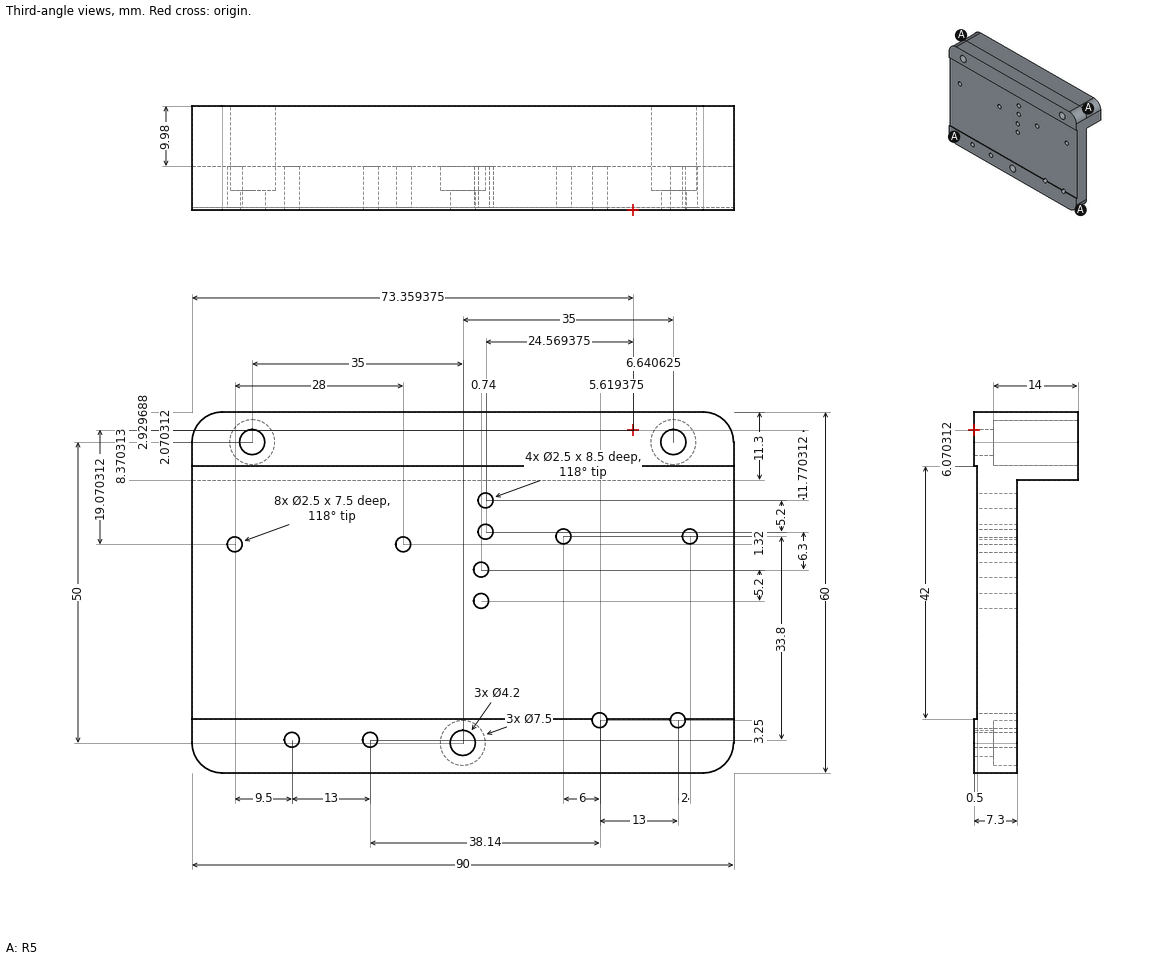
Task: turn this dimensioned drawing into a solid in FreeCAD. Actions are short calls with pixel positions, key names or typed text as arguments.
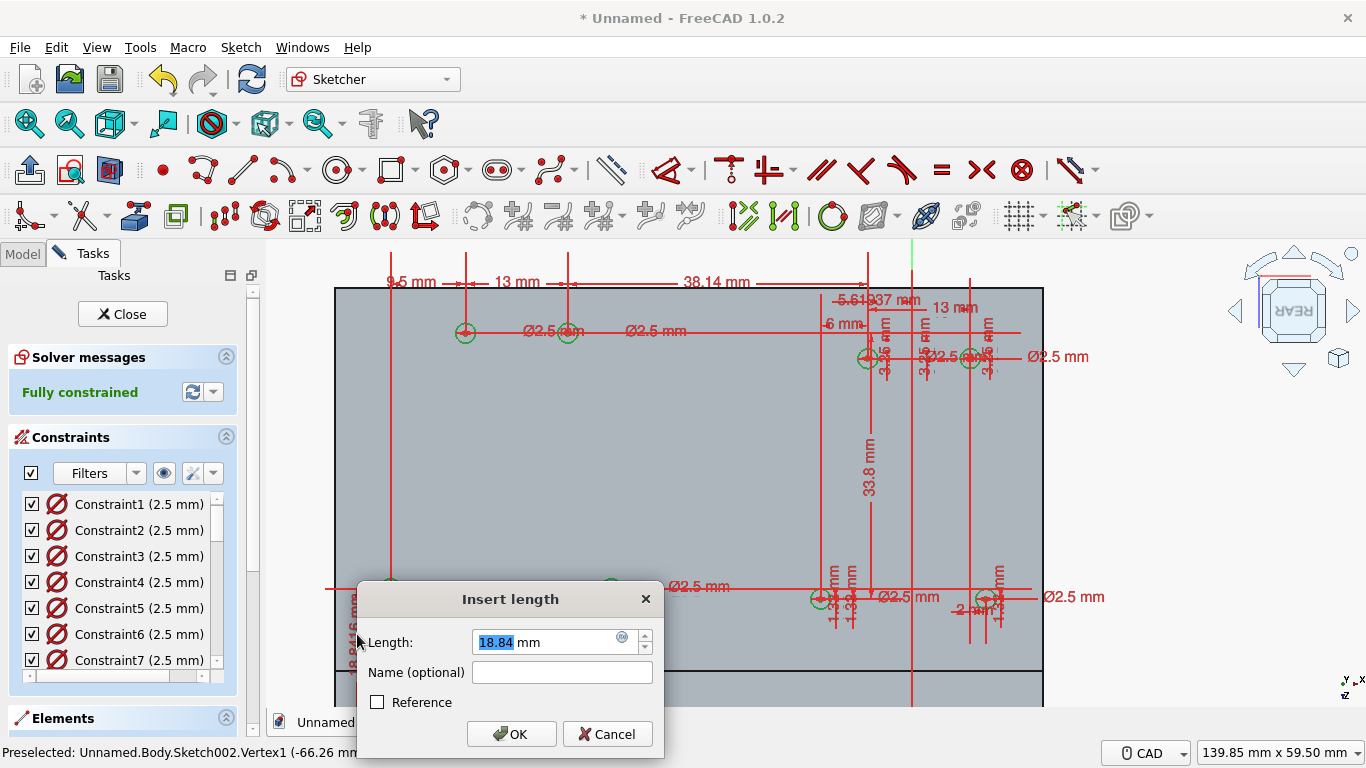
text(19.070312)
key(Return)
key(Escape)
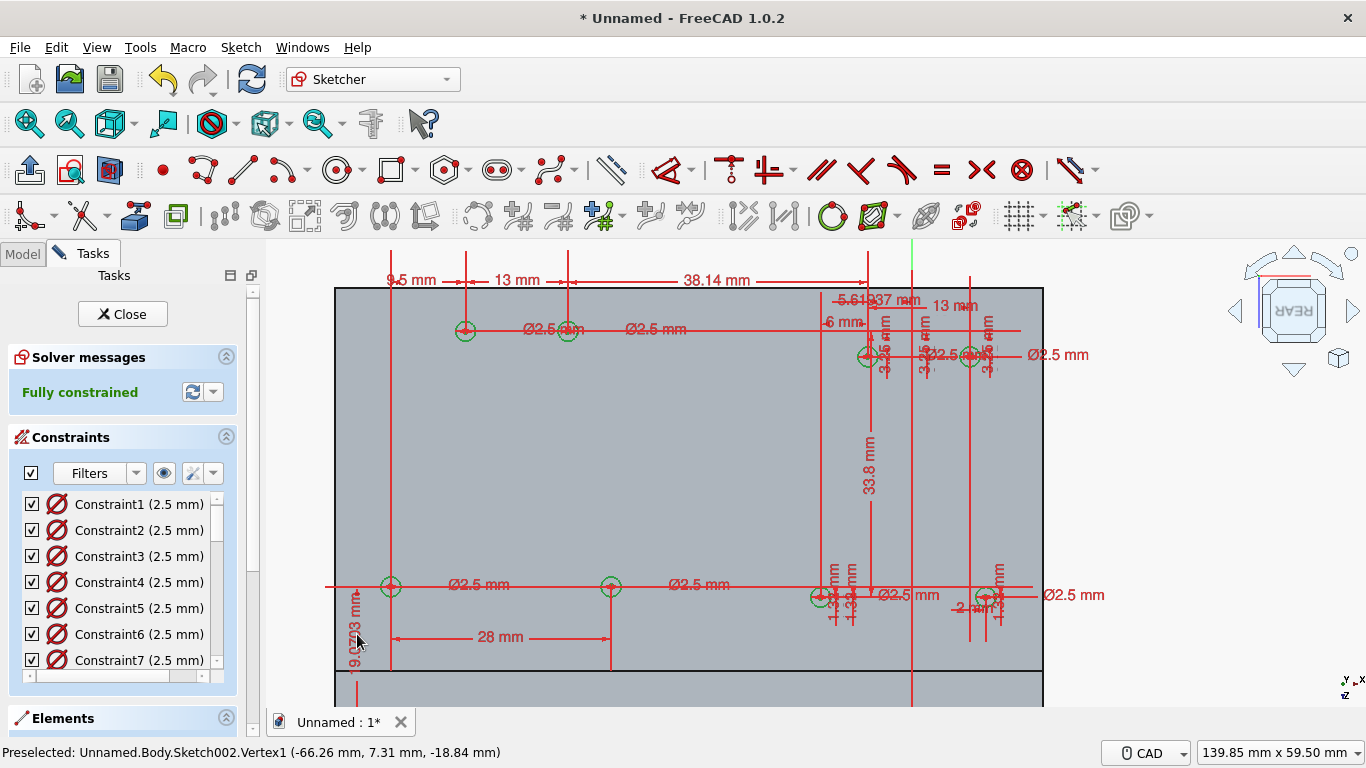
click(123, 314)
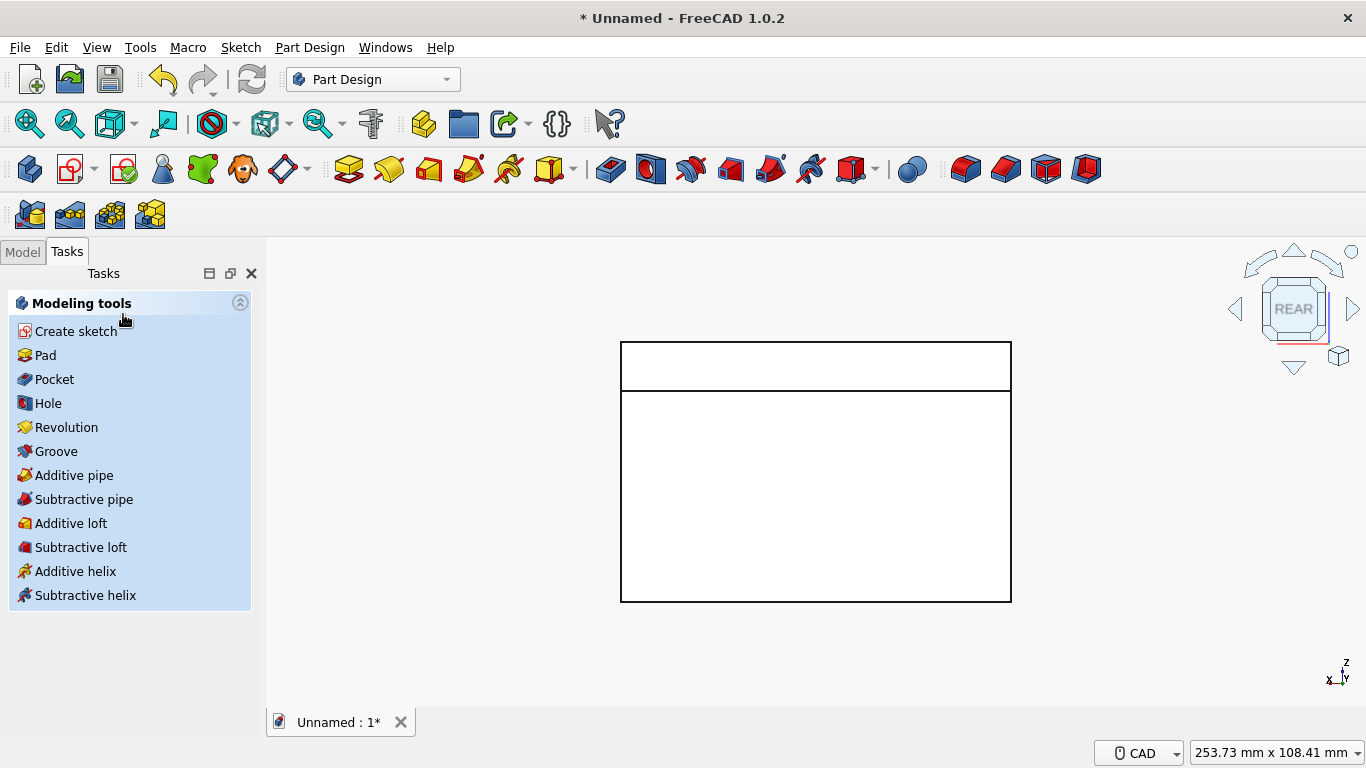
click(652, 170)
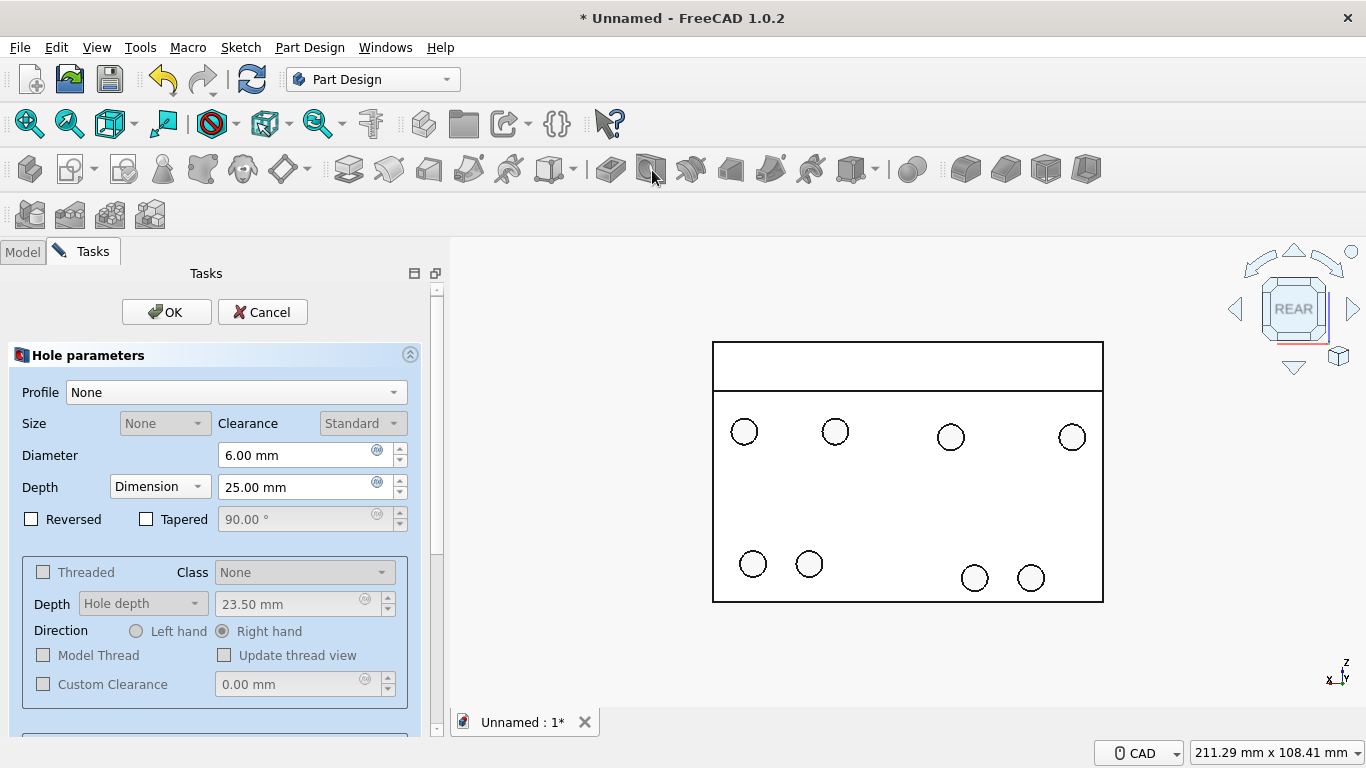
triple_click(305, 455)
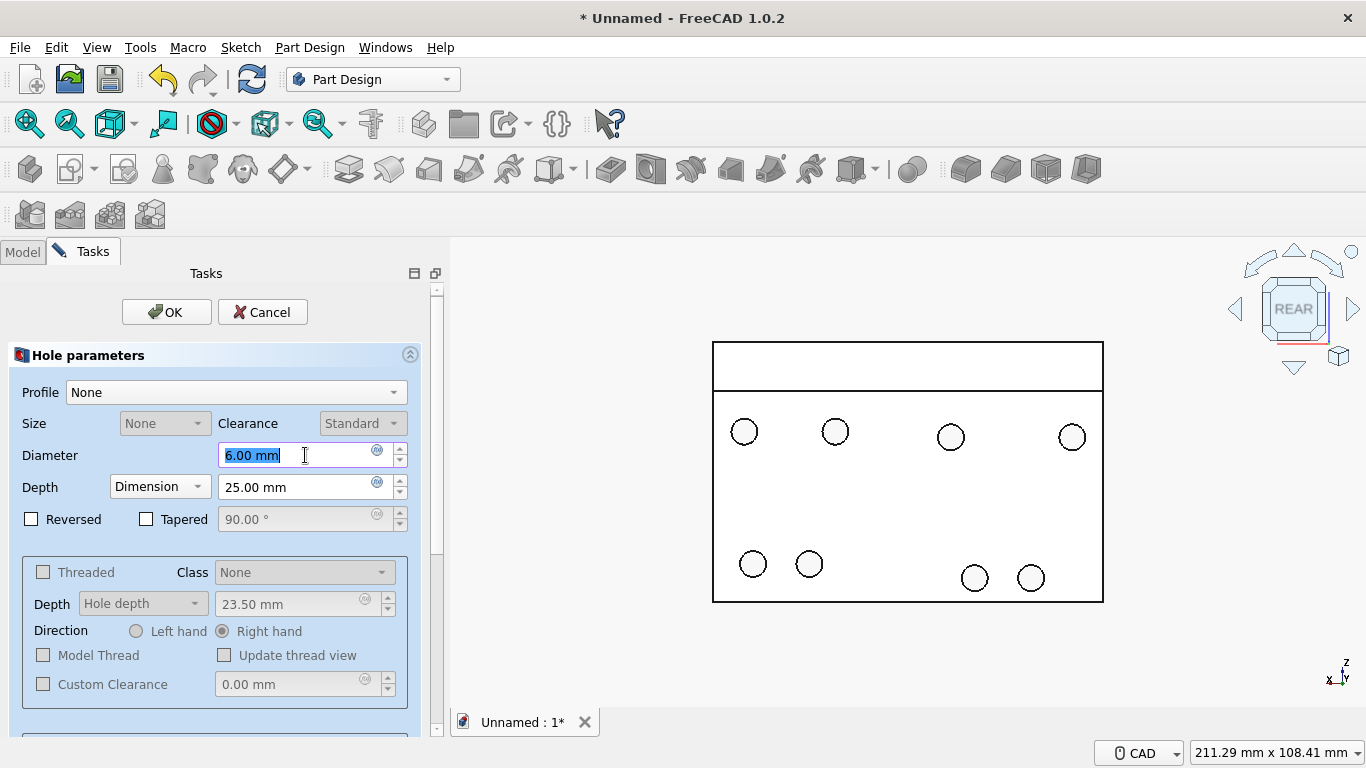
text(2.5)
key(Tab)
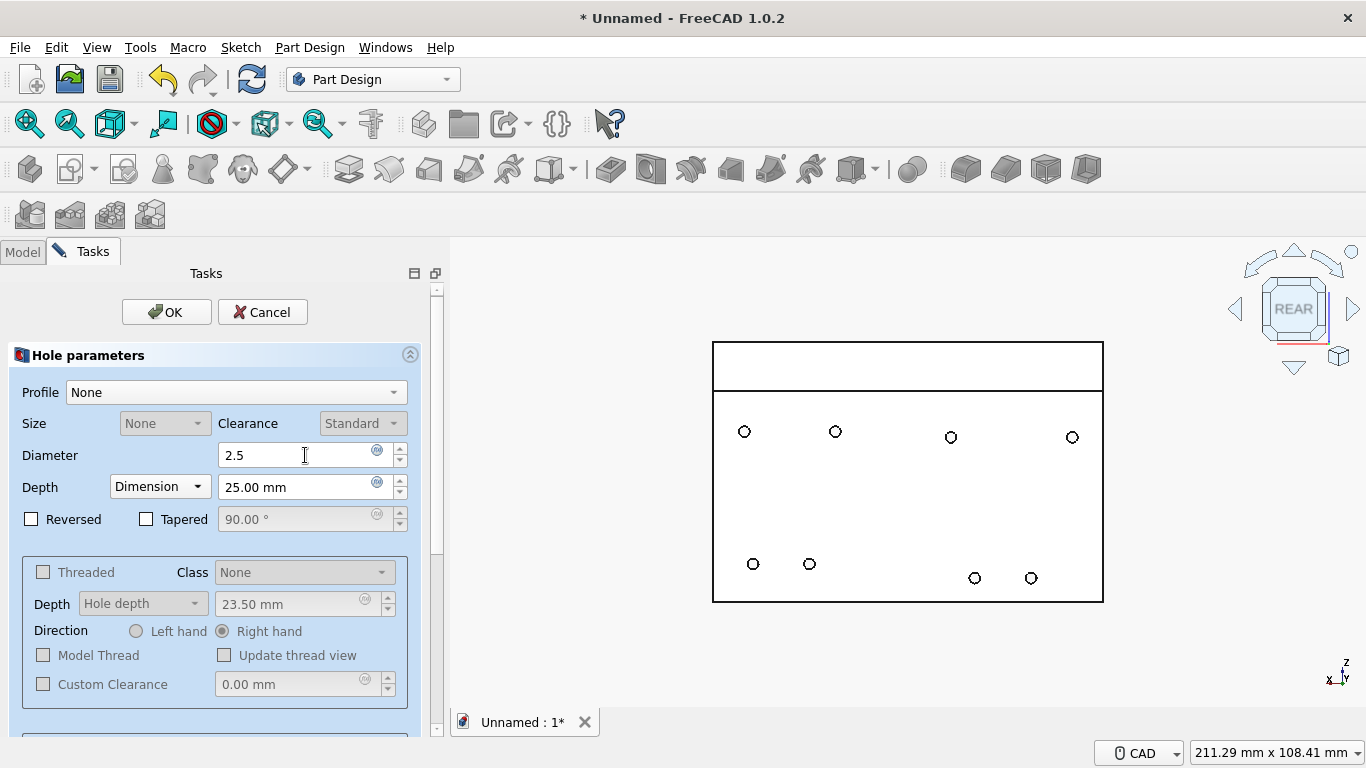
triple_click(305, 487)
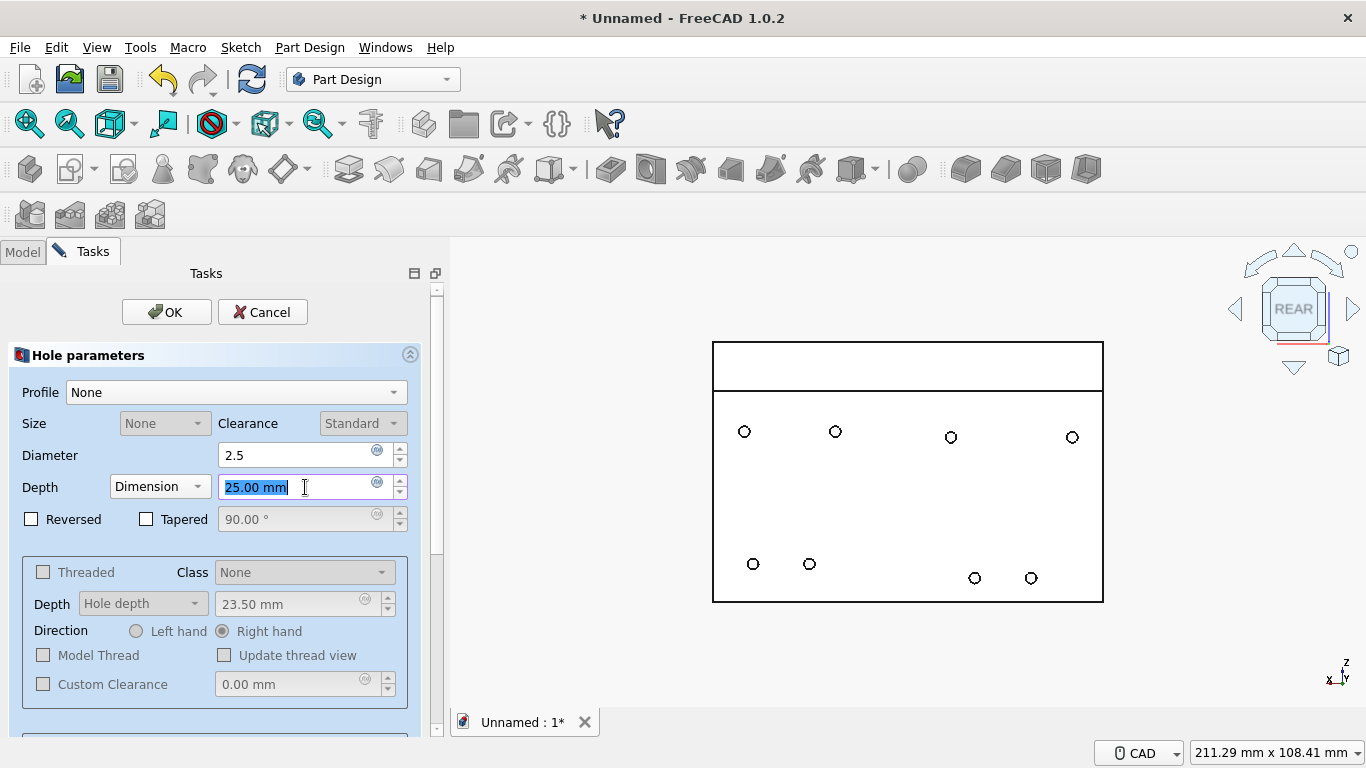
text(7.5)
key(Tab)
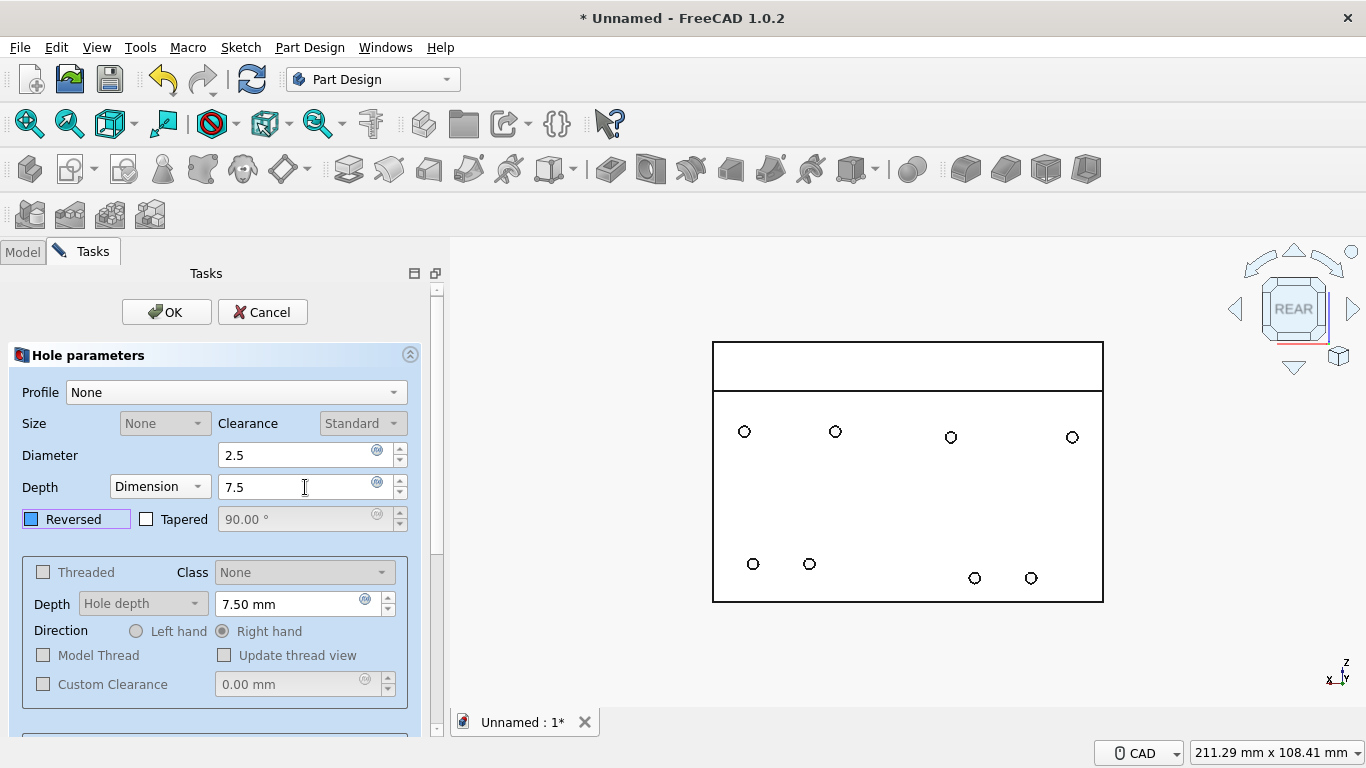
click(167, 312)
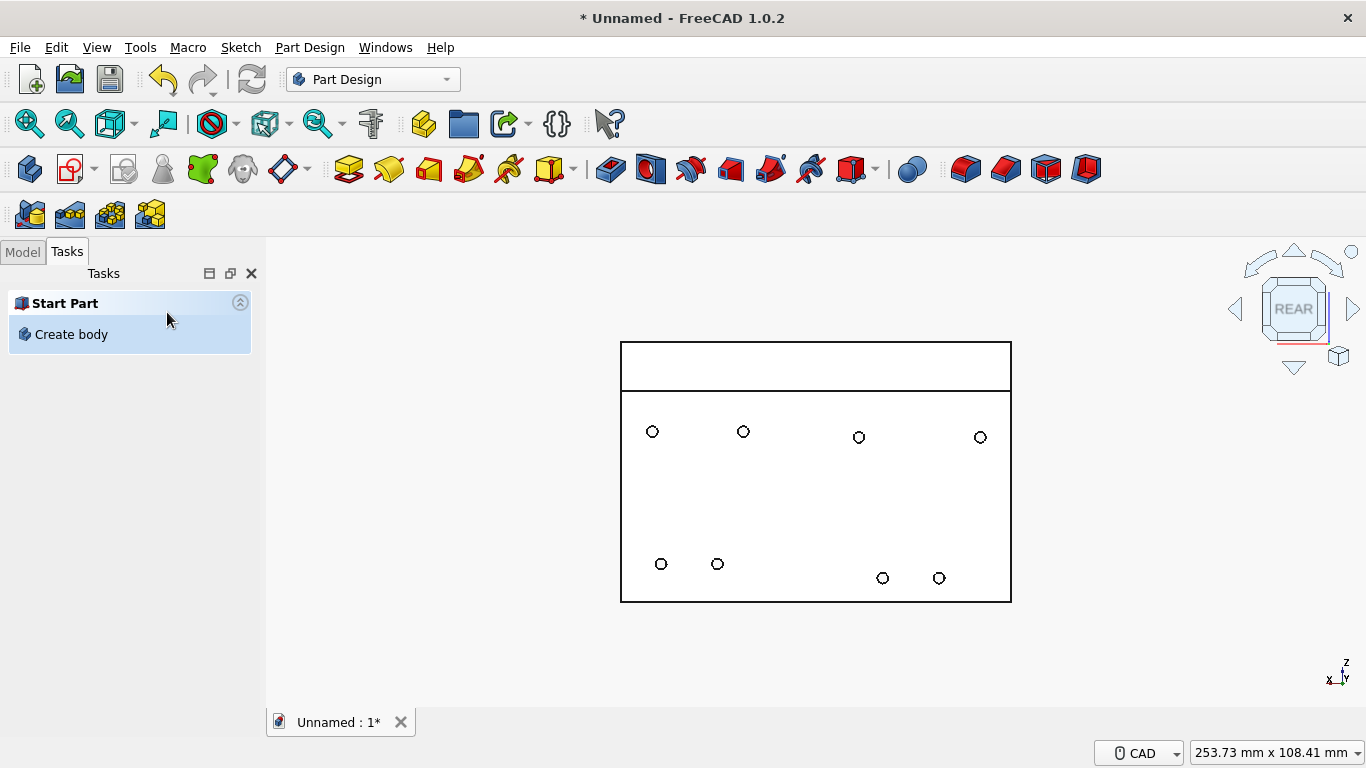
key(0)